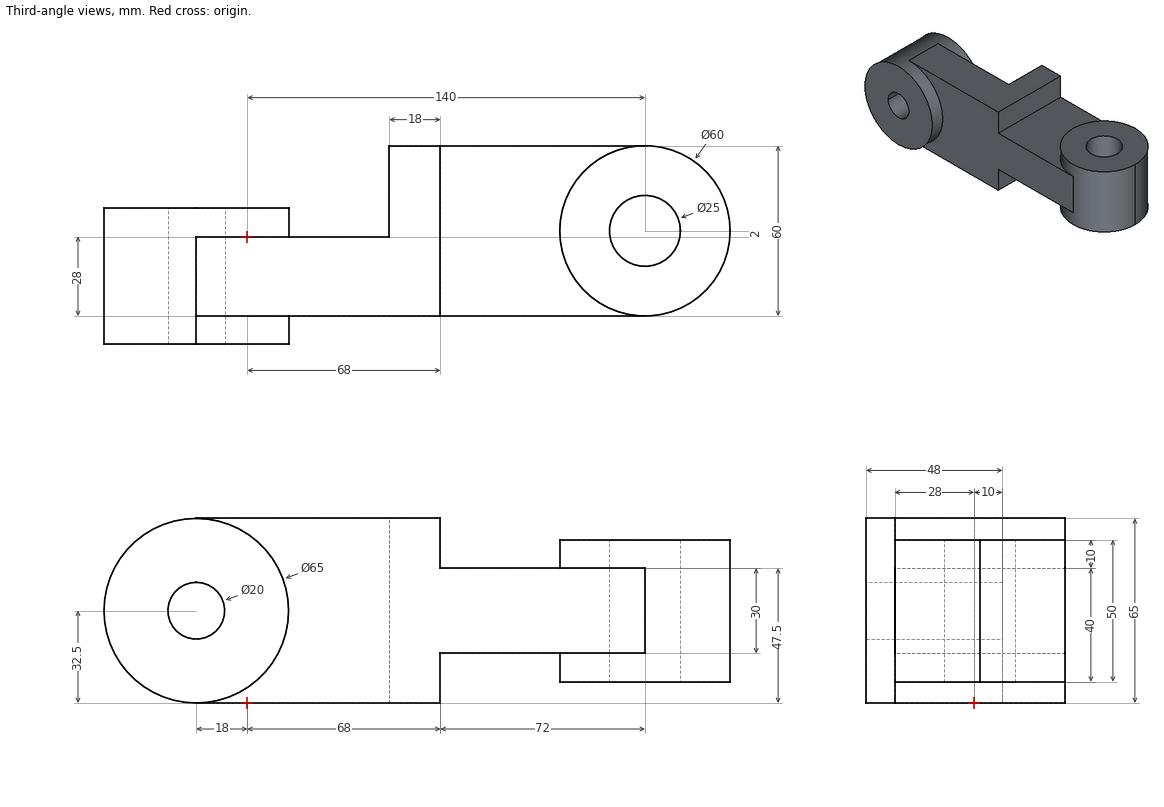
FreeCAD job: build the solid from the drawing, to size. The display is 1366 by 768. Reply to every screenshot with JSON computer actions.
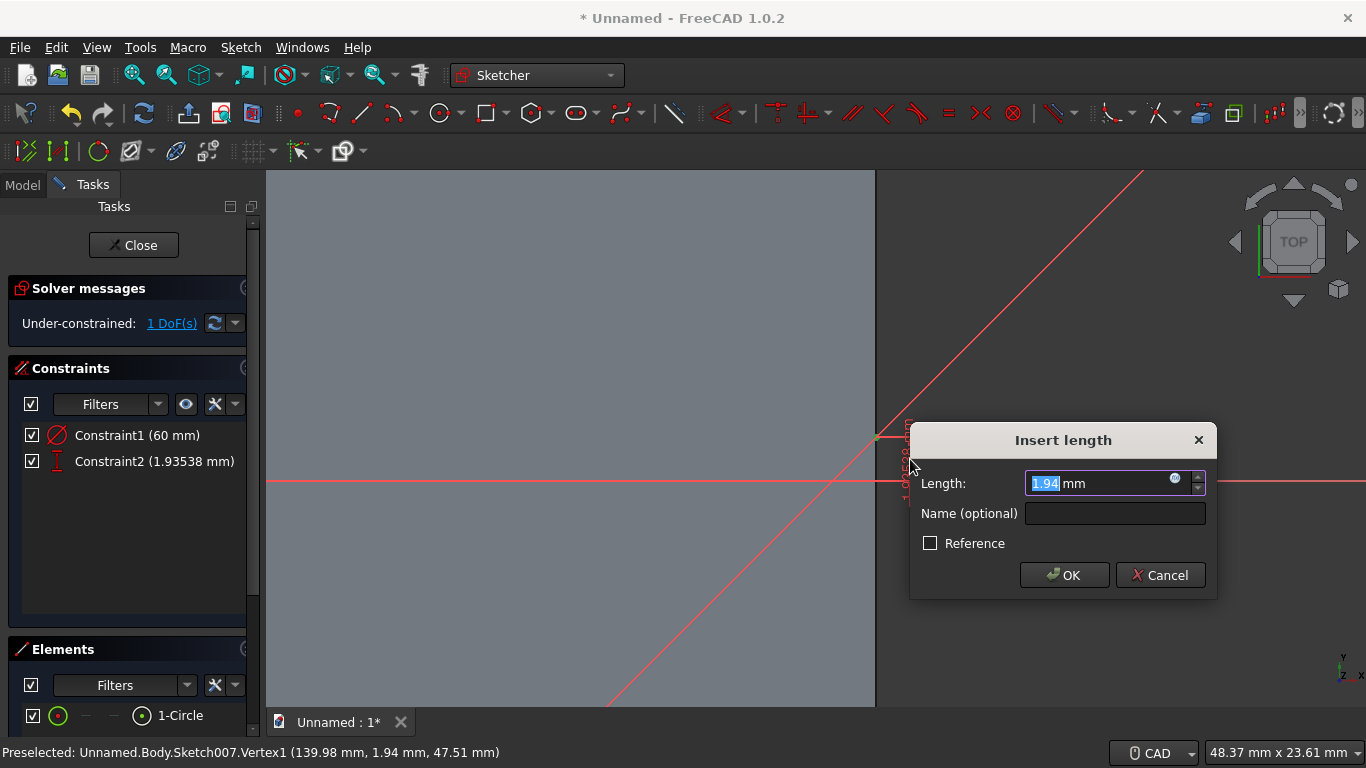
{"action": "type", "text": "2"}
{"action": "key", "text": "Return"}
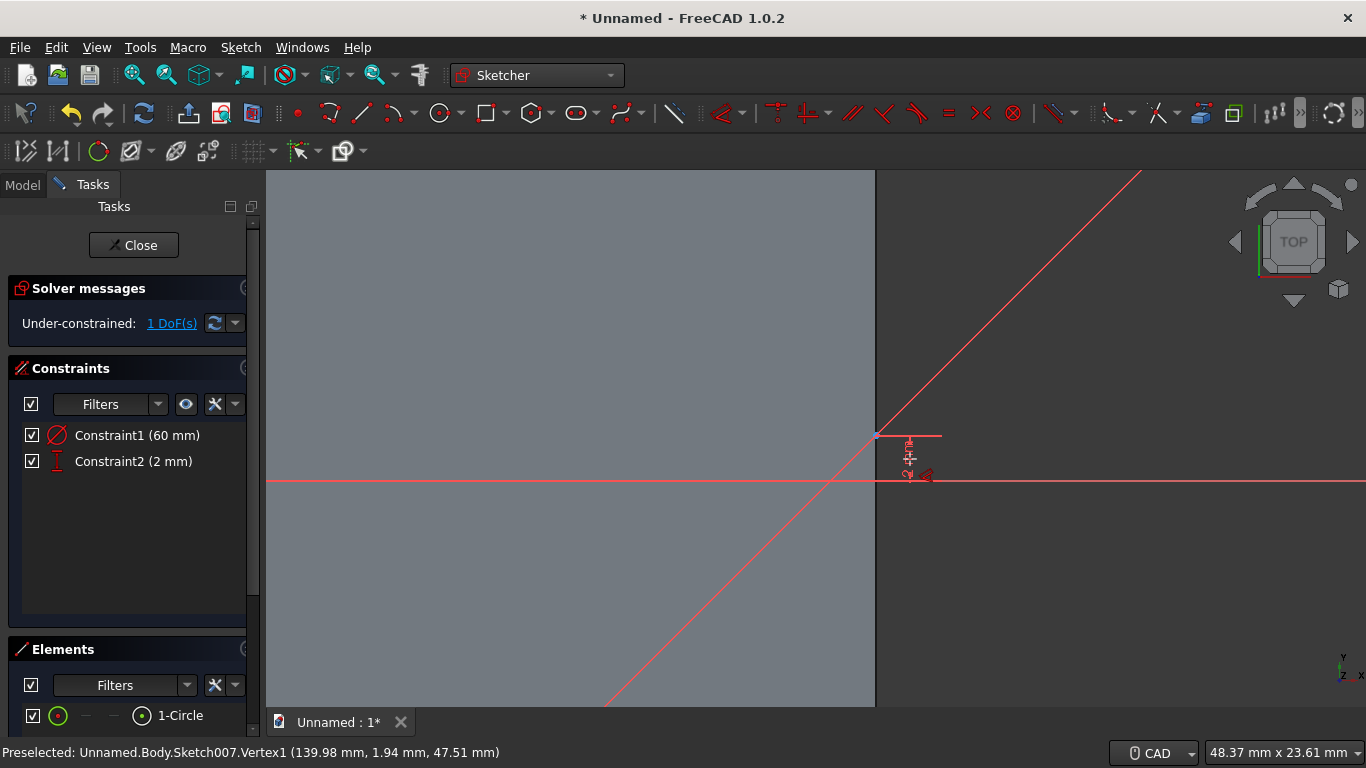
{"action": "scroll", "coordinate": [705, 439], "scroll_direction": "down", "scroll_amount": 7}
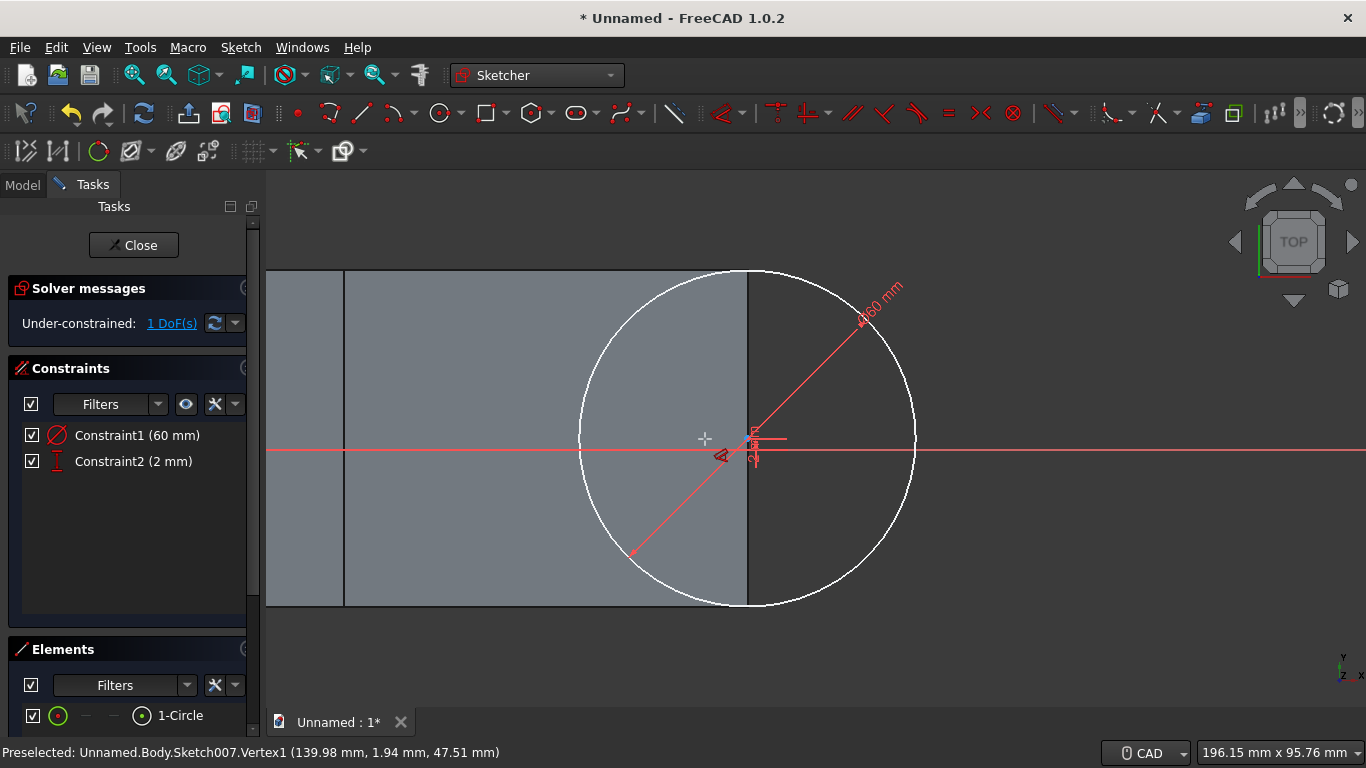
{"action": "left_click", "coordinate": [747, 439]}
{"action": "left_click", "coordinate": [521, 484]}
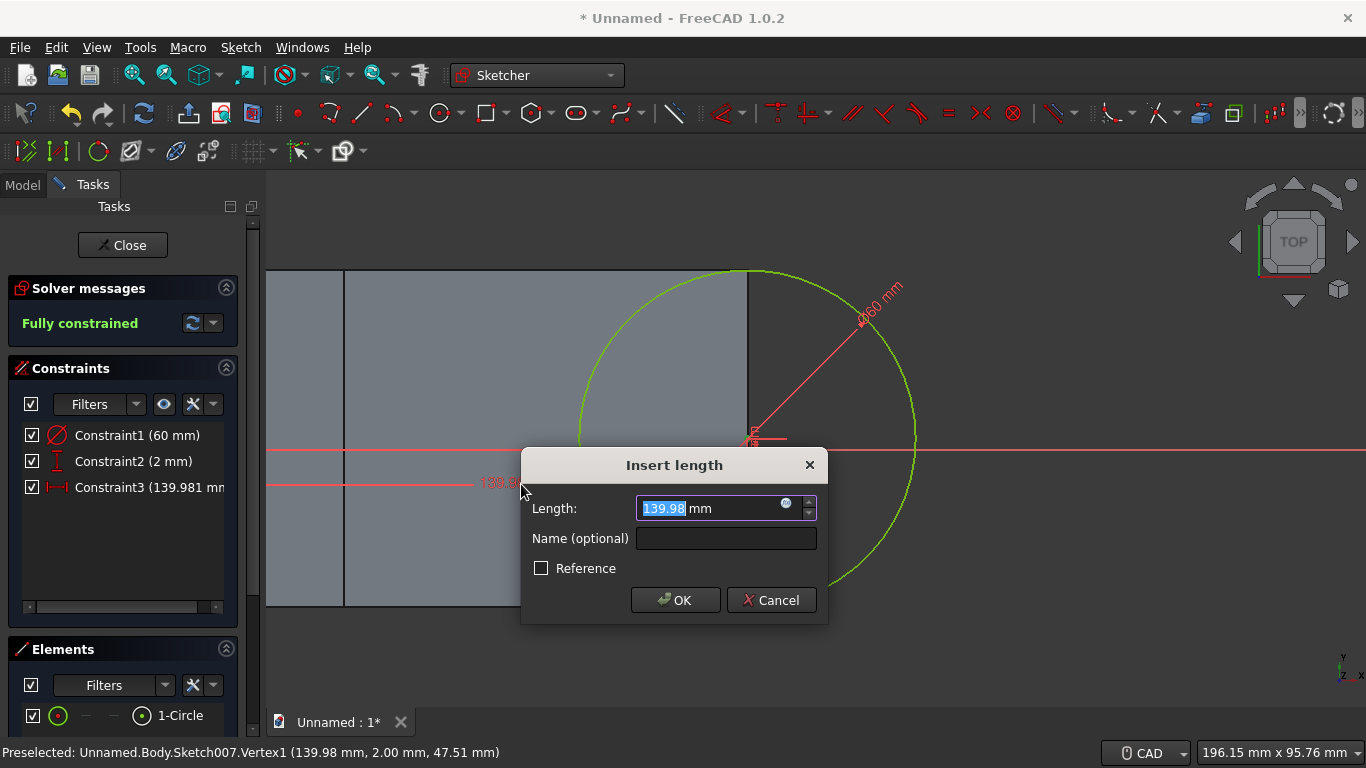
{"action": "type", "text": "140"}
{"action": "key", "text": "Return"}
{"action": "key", "text": "Escape"}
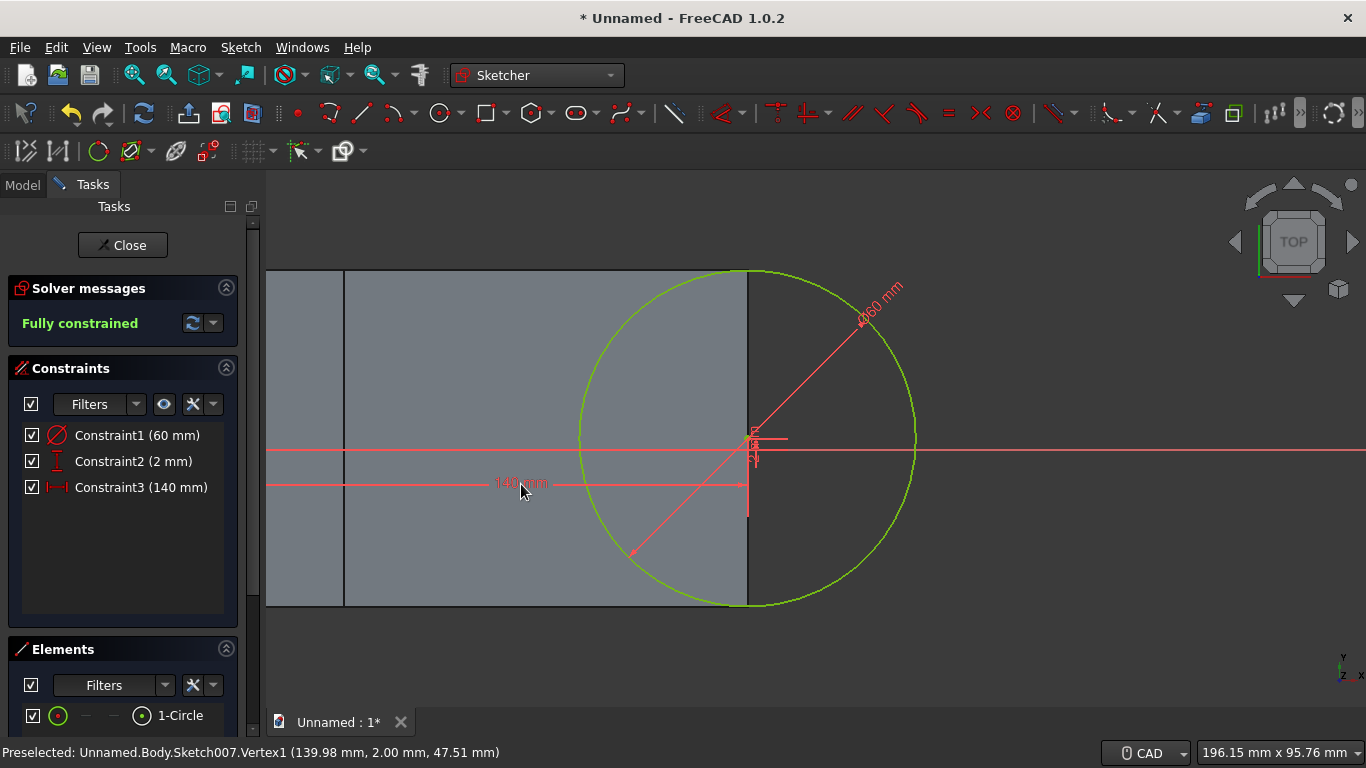
{"action": "left_click", "coordinate": [123, 245]}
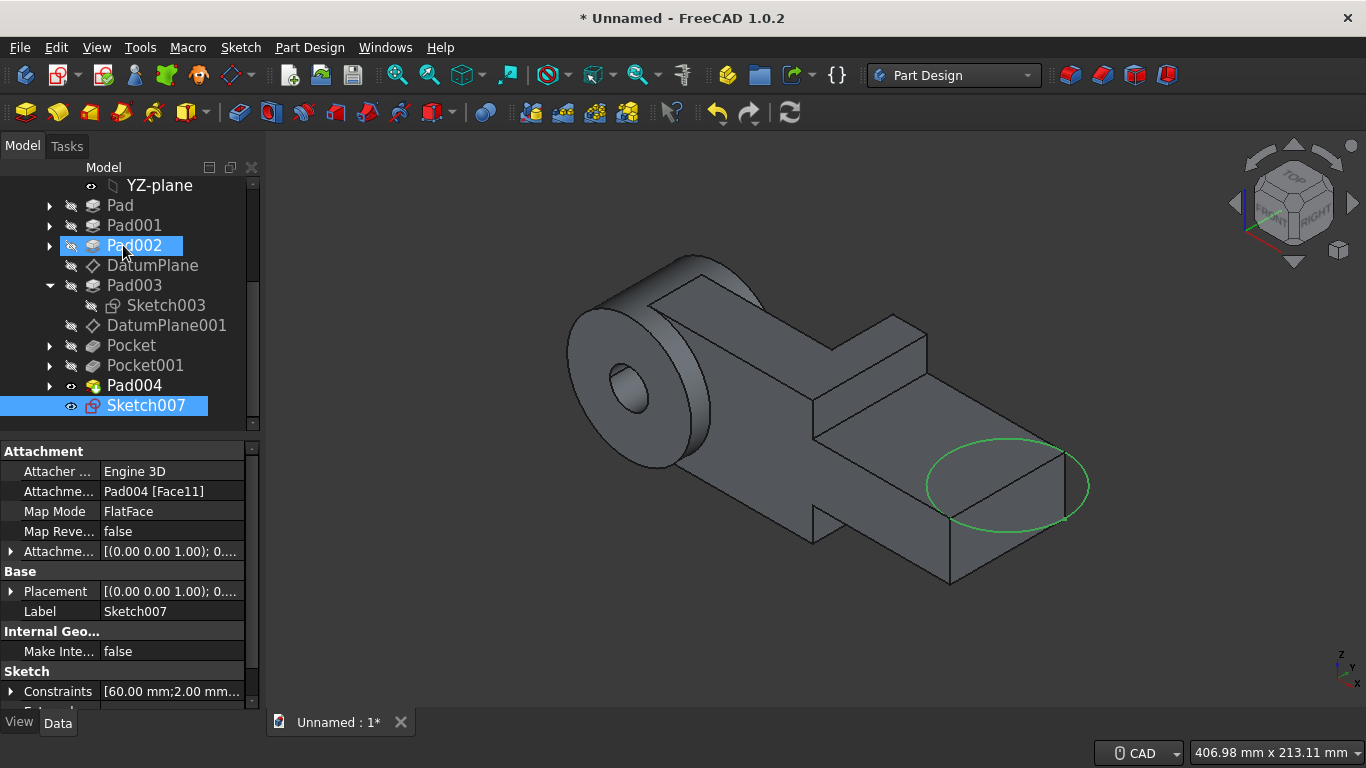
{"action": "left_click", "coordinate": [26, 112]}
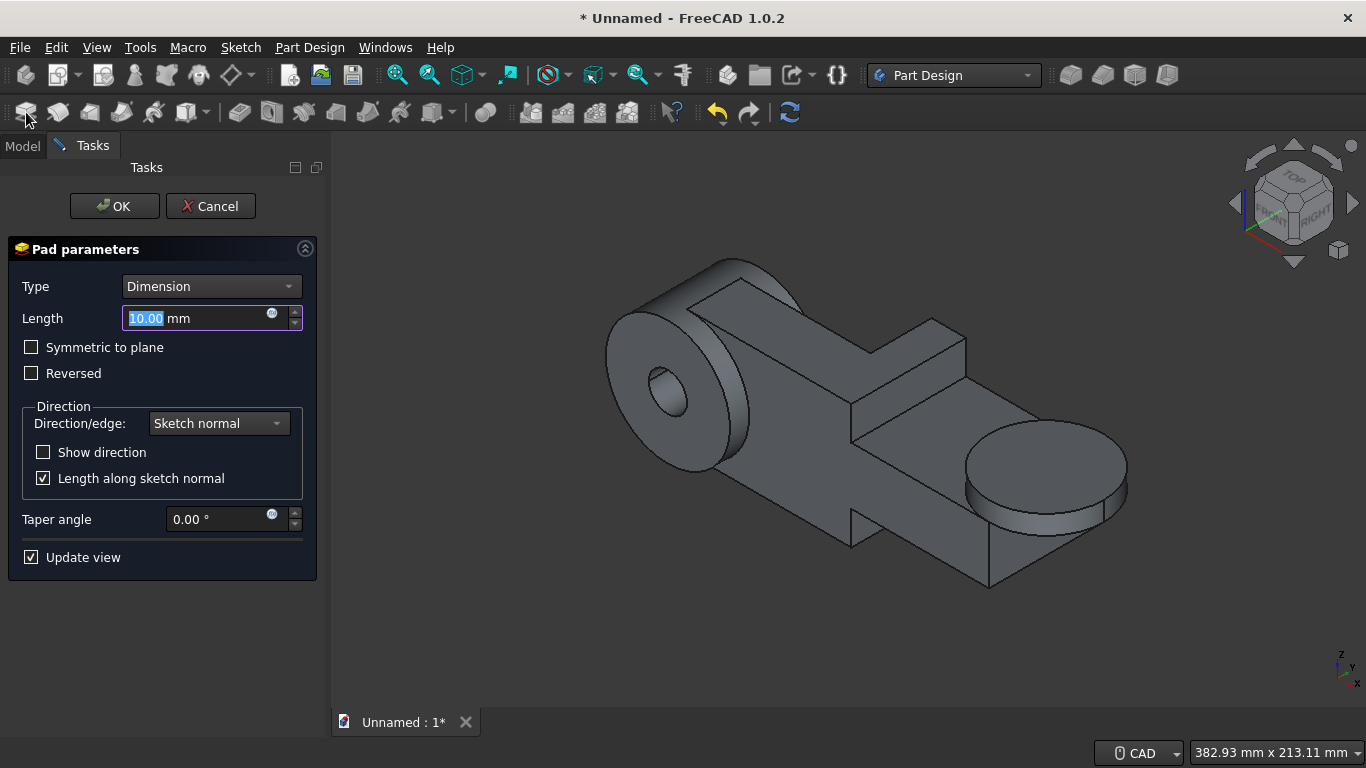
{"action": "type", "text": "40"}
{"action": "key", "text": "Tab"}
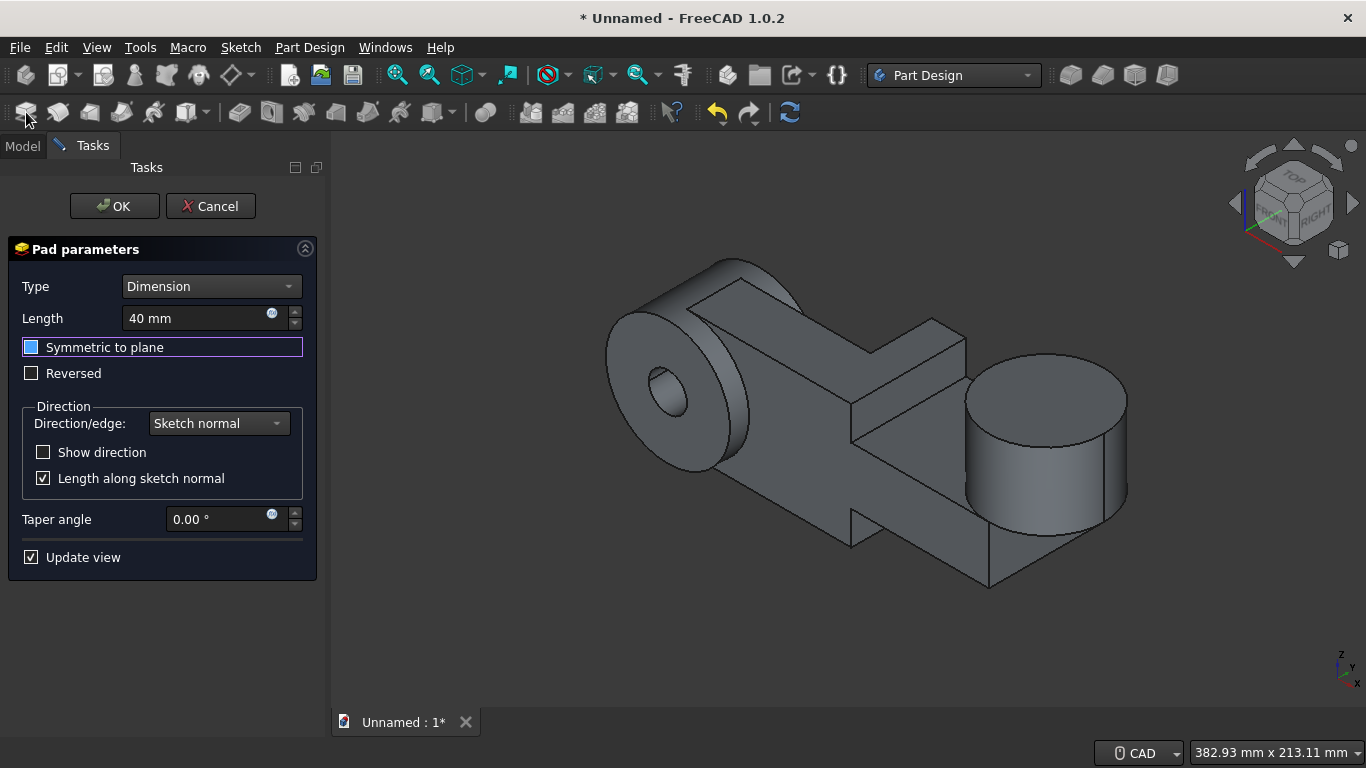
{"action": "left_click", "coordinate": [30, 373]}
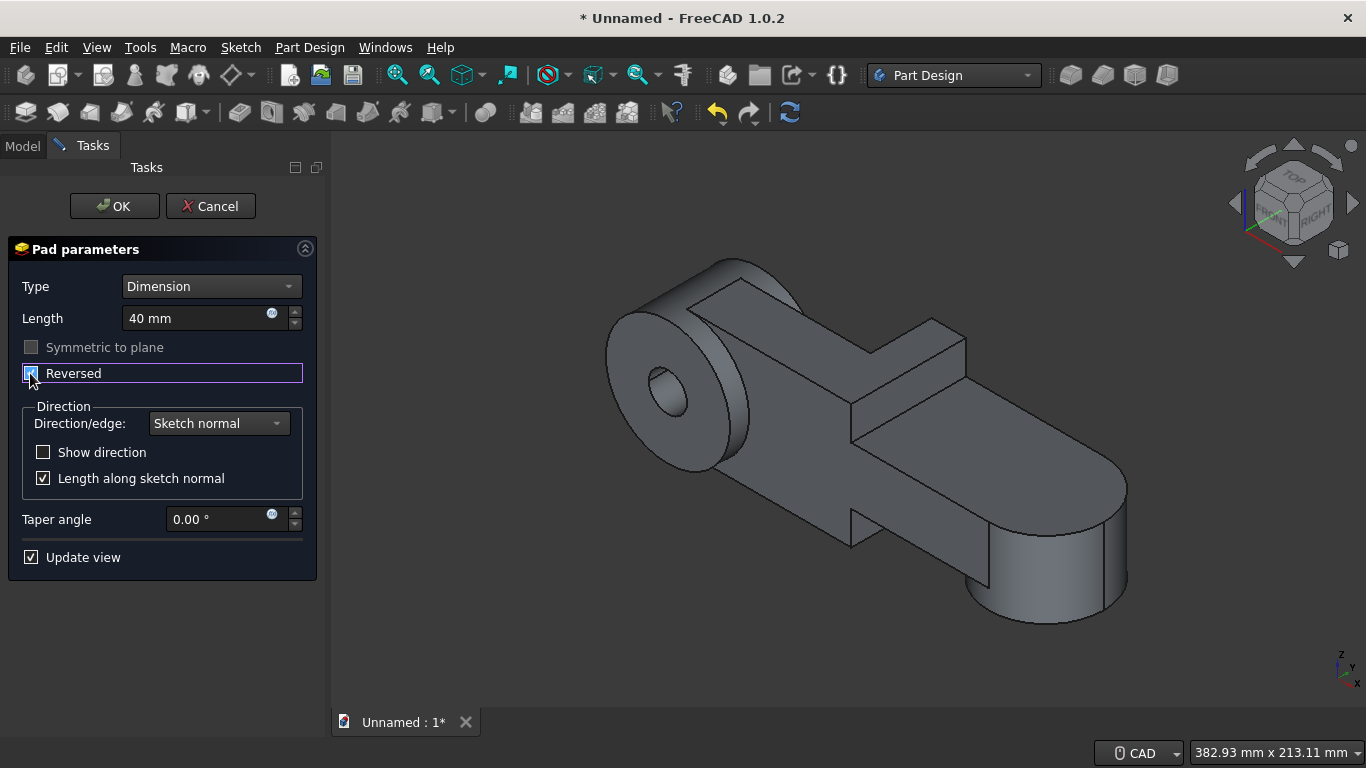
{"action": "left_click", "coordinate": [115, 206]}